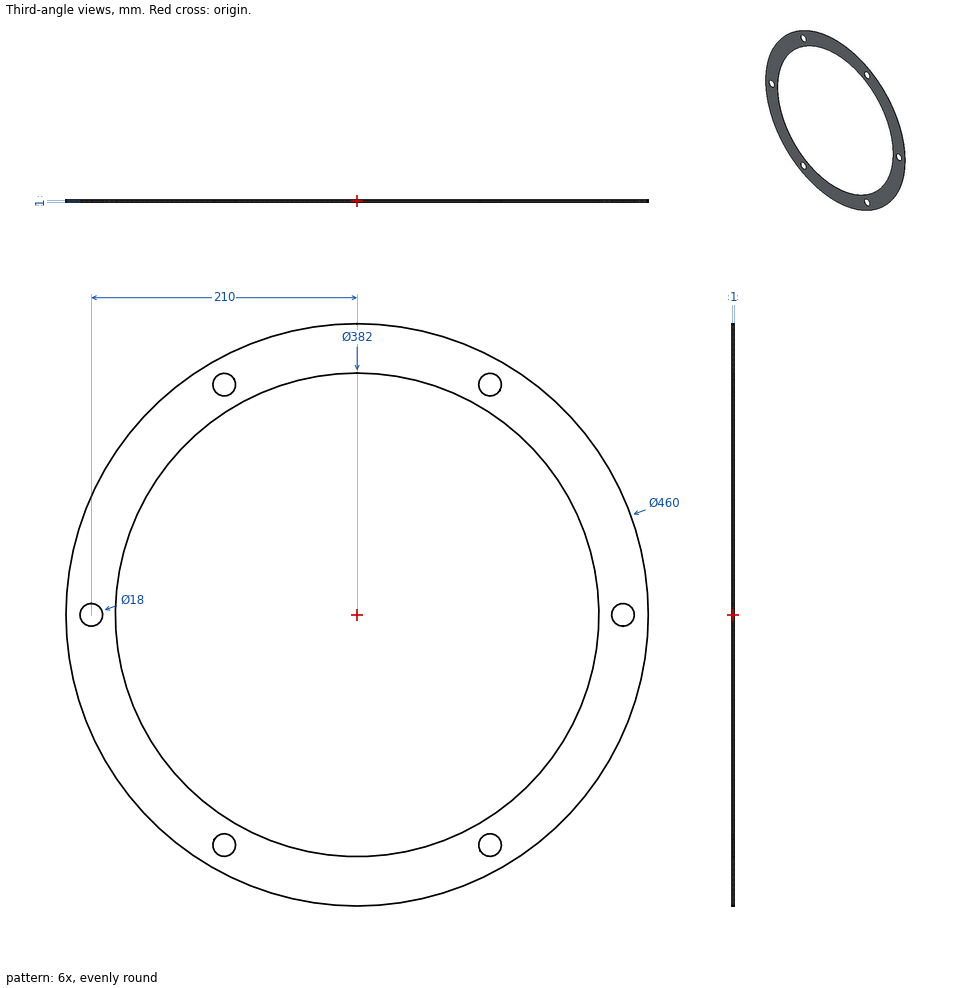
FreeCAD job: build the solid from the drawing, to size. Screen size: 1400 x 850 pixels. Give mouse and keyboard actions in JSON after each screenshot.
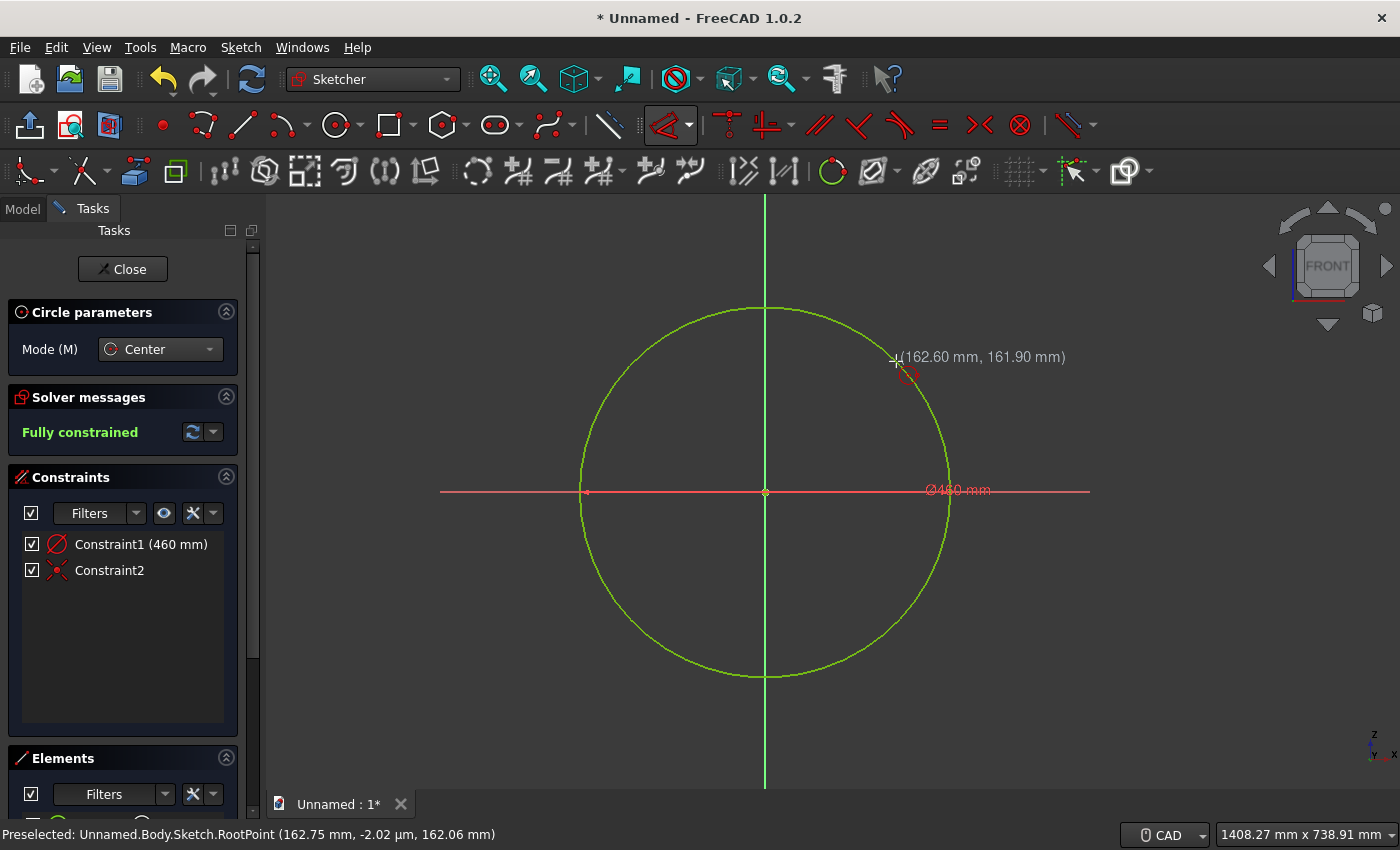
{"action": "left_click", "coordinate": [765, 492]}
{"action": "mouse_move", "coordinate": [874, 384]}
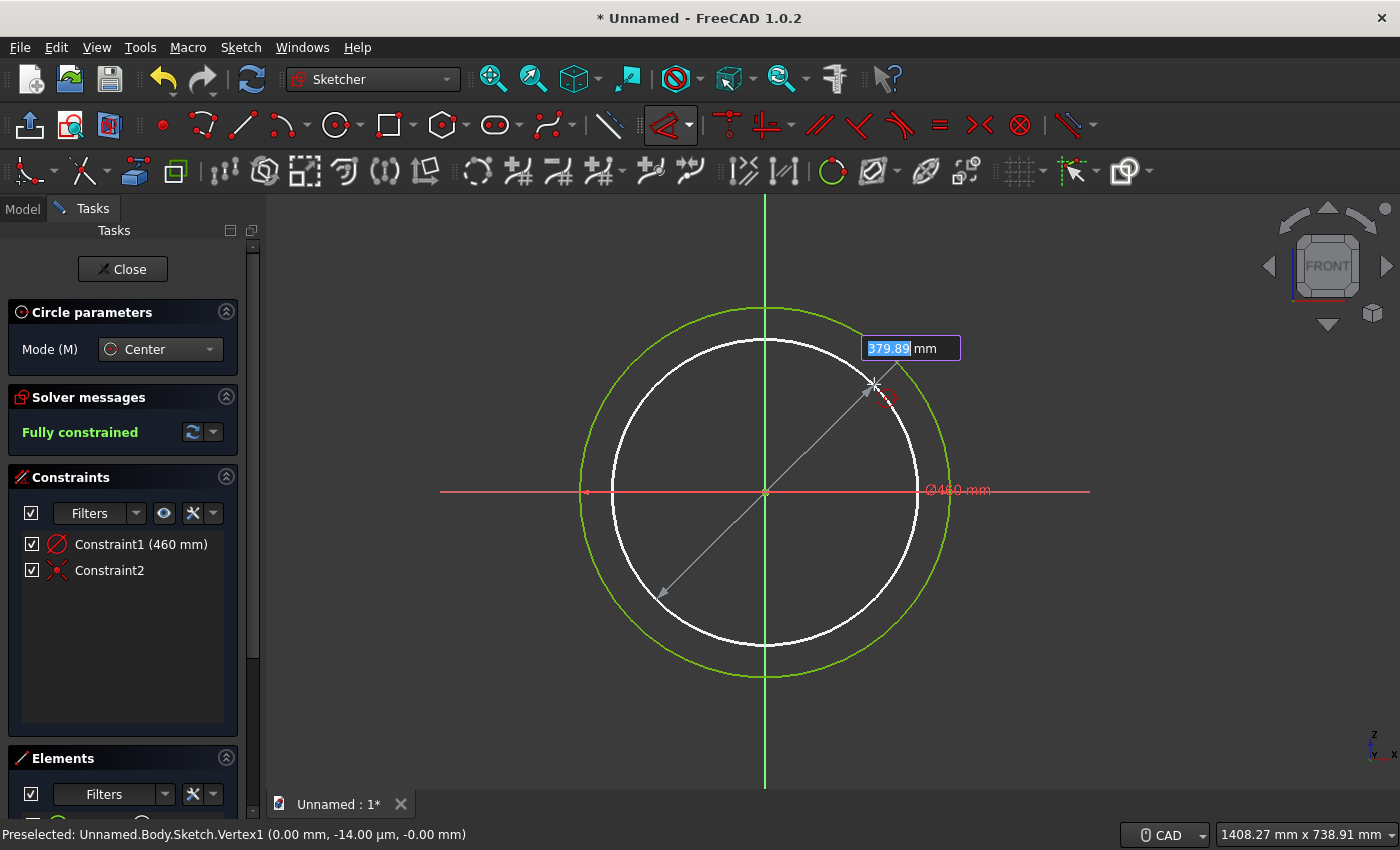
{"action": "type", "text": "382"}
{"action": "key", "text": "Return"}
{"action": "key", "text": "Escape"}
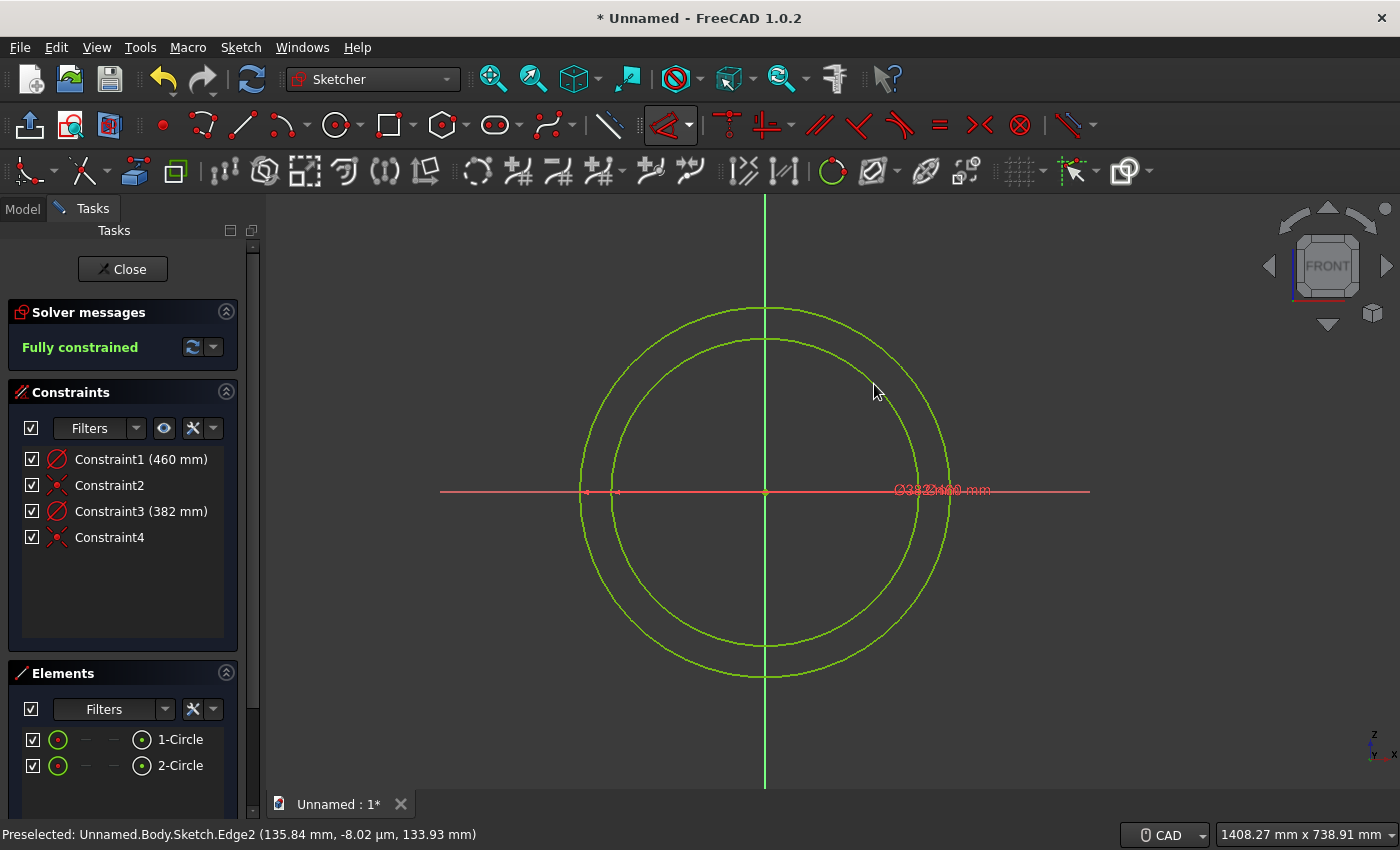
{"action": "left_click", "coordinate": [123, 269]}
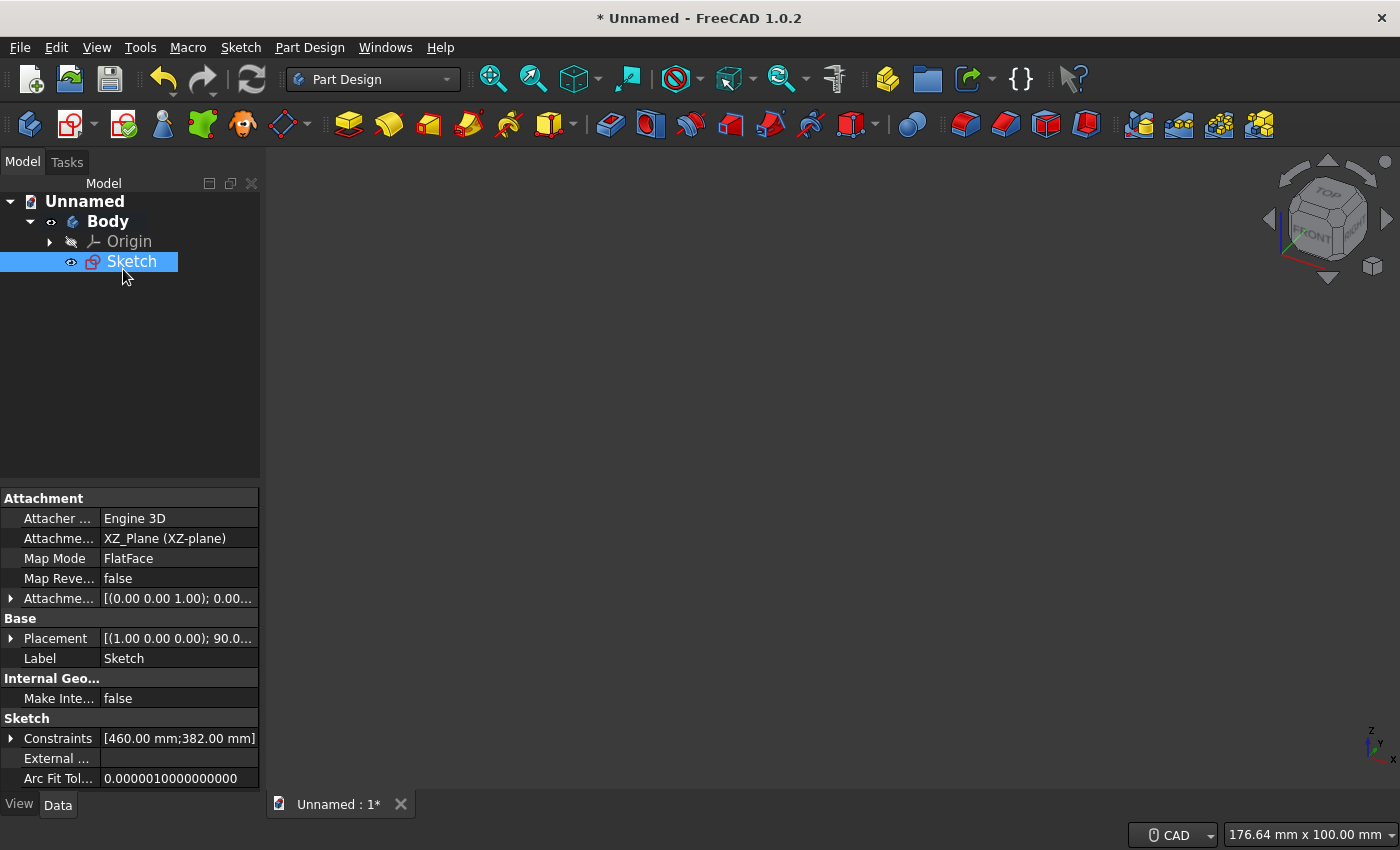
{"action": "left_click", "coordinate": [350, 124]}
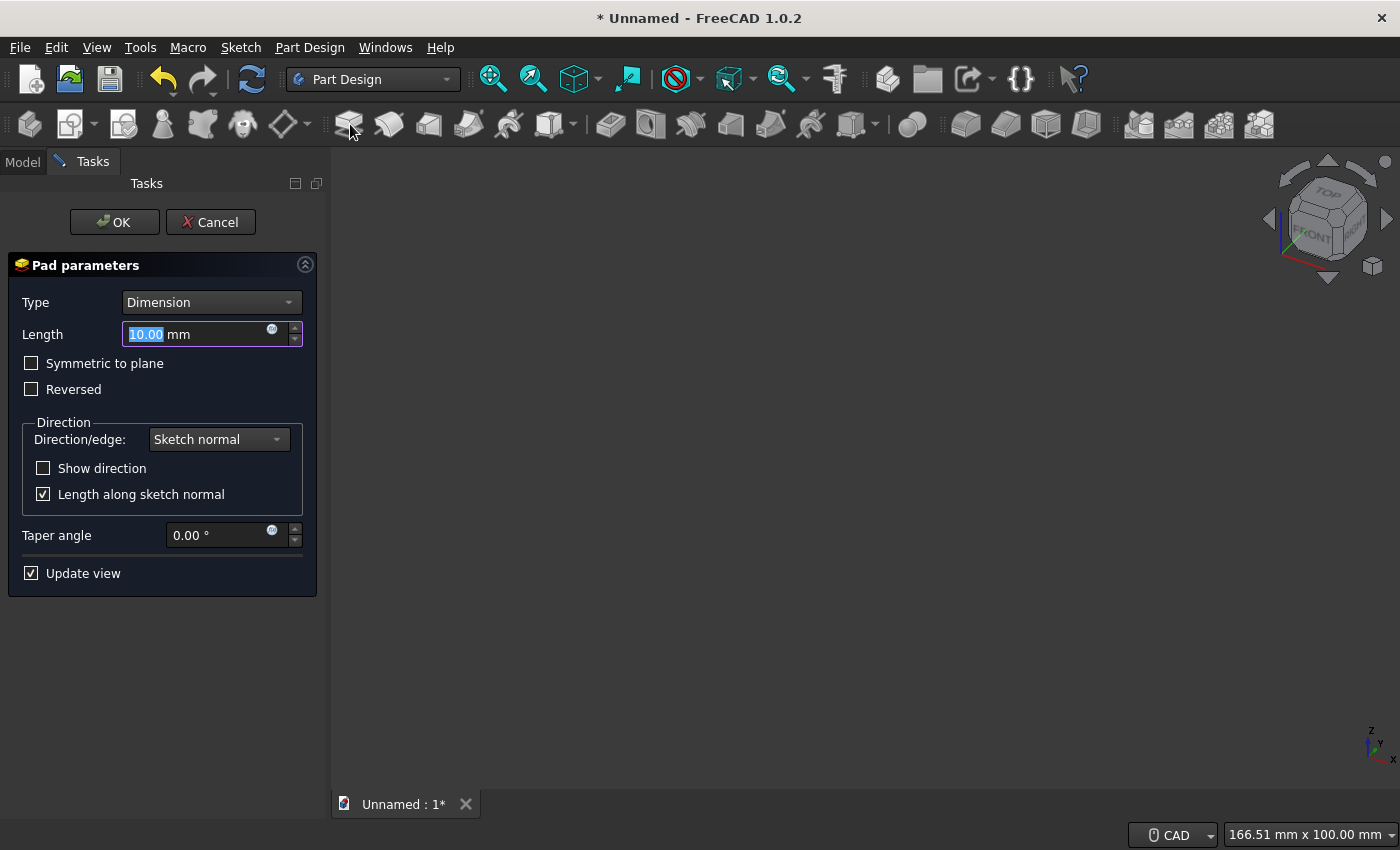
{"action": "type", "text": "1"}
{"action": "key", "text": "Tab"}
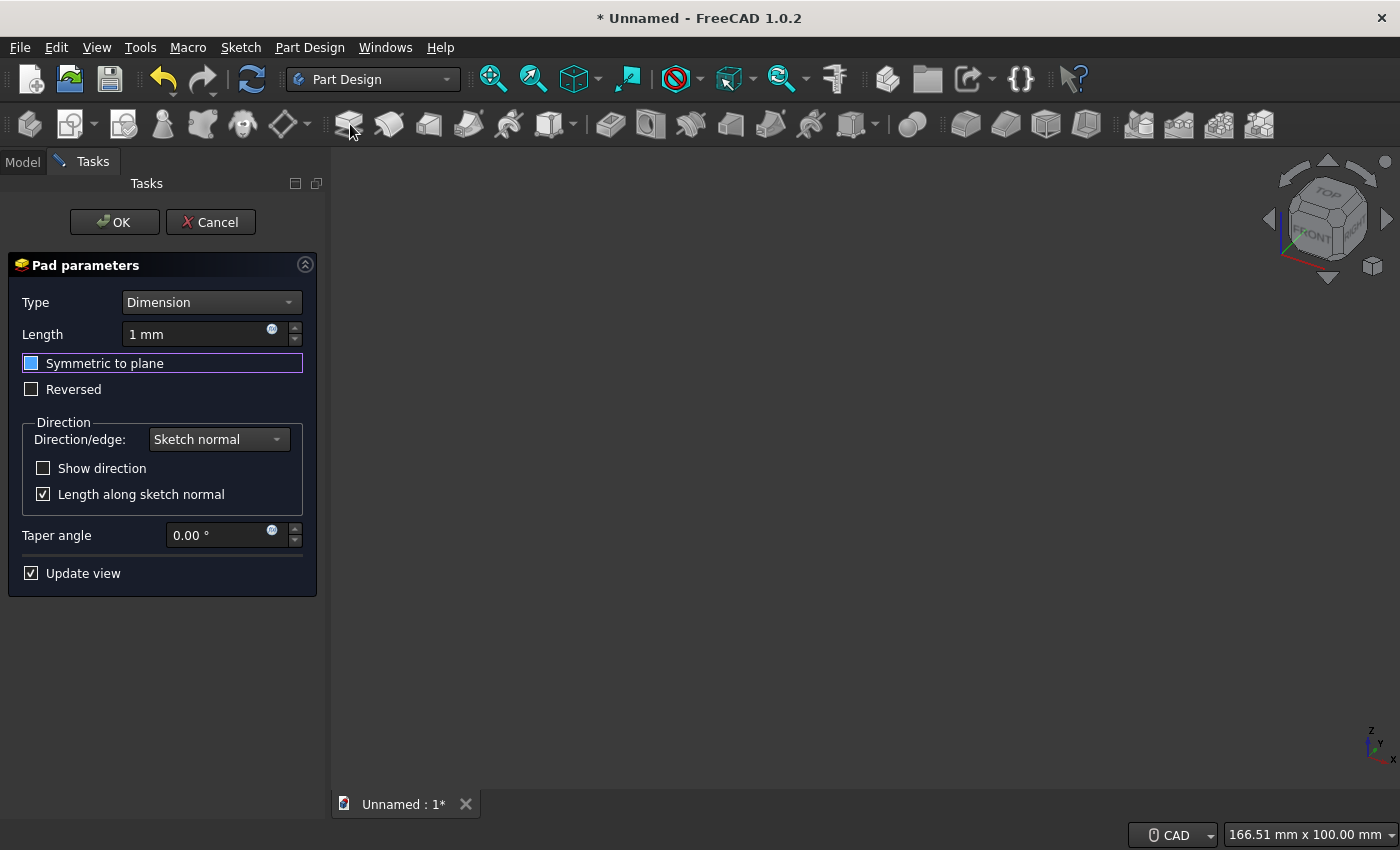
{"action": "left_click", "coordinate": [30, 363]}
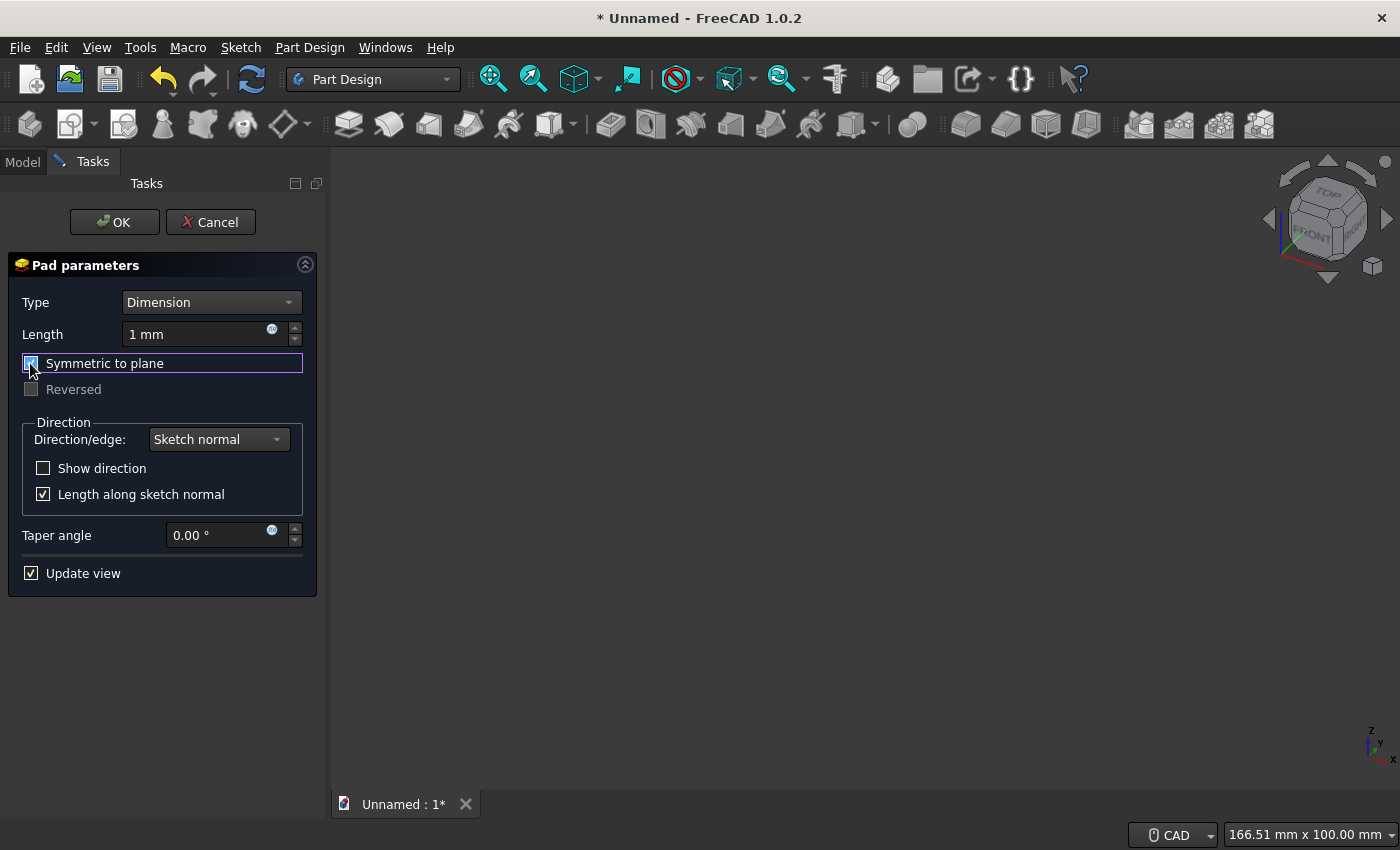
{"action": "left_click", "coordinate": [115, 222]}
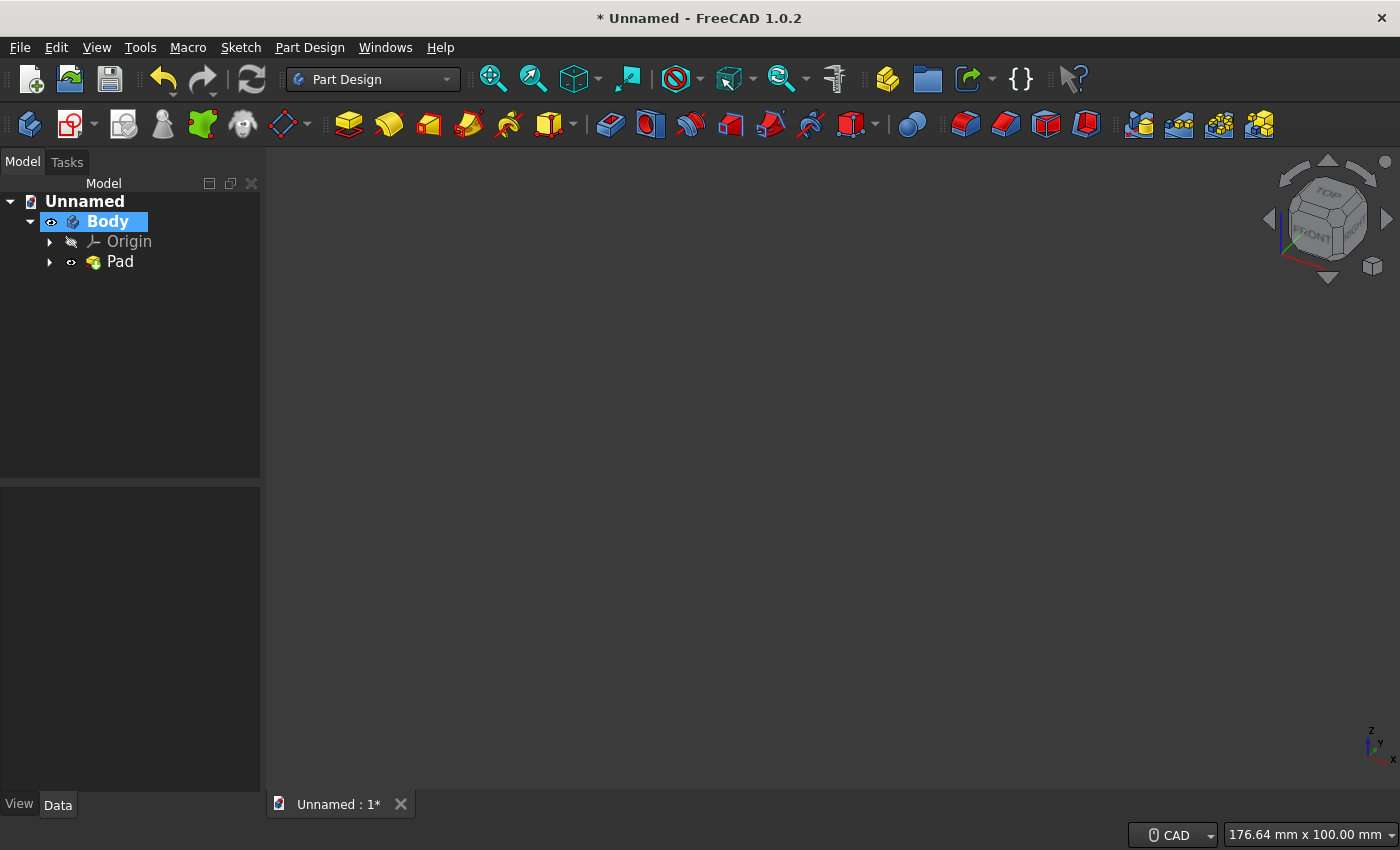
{"action": "key", "text": "v f"}